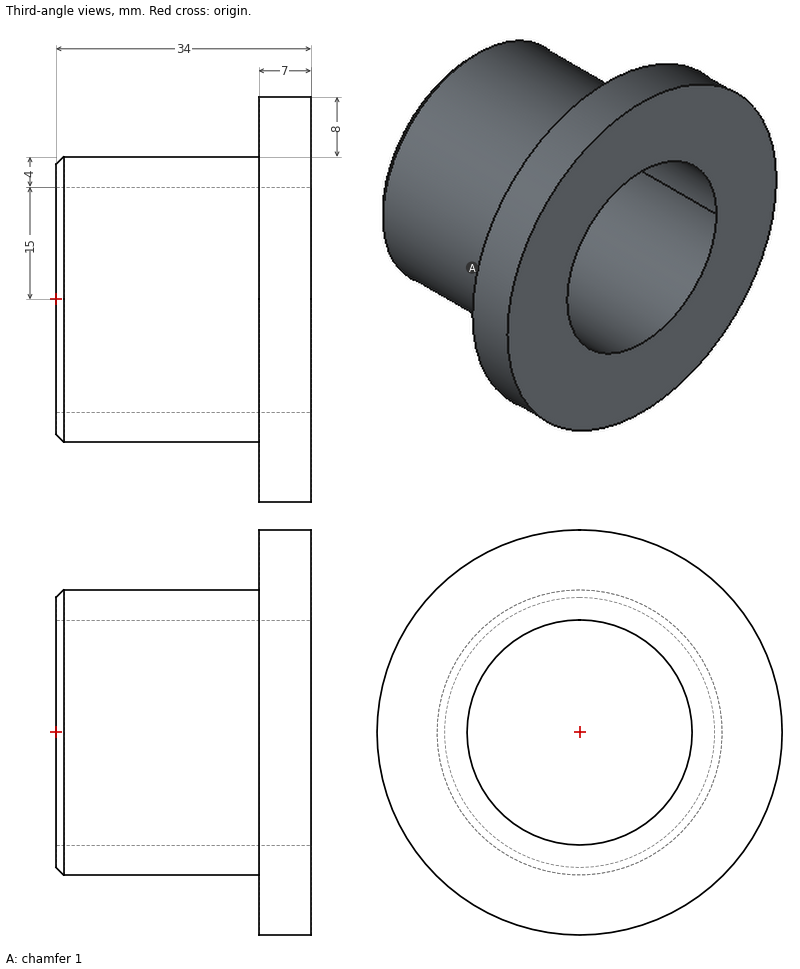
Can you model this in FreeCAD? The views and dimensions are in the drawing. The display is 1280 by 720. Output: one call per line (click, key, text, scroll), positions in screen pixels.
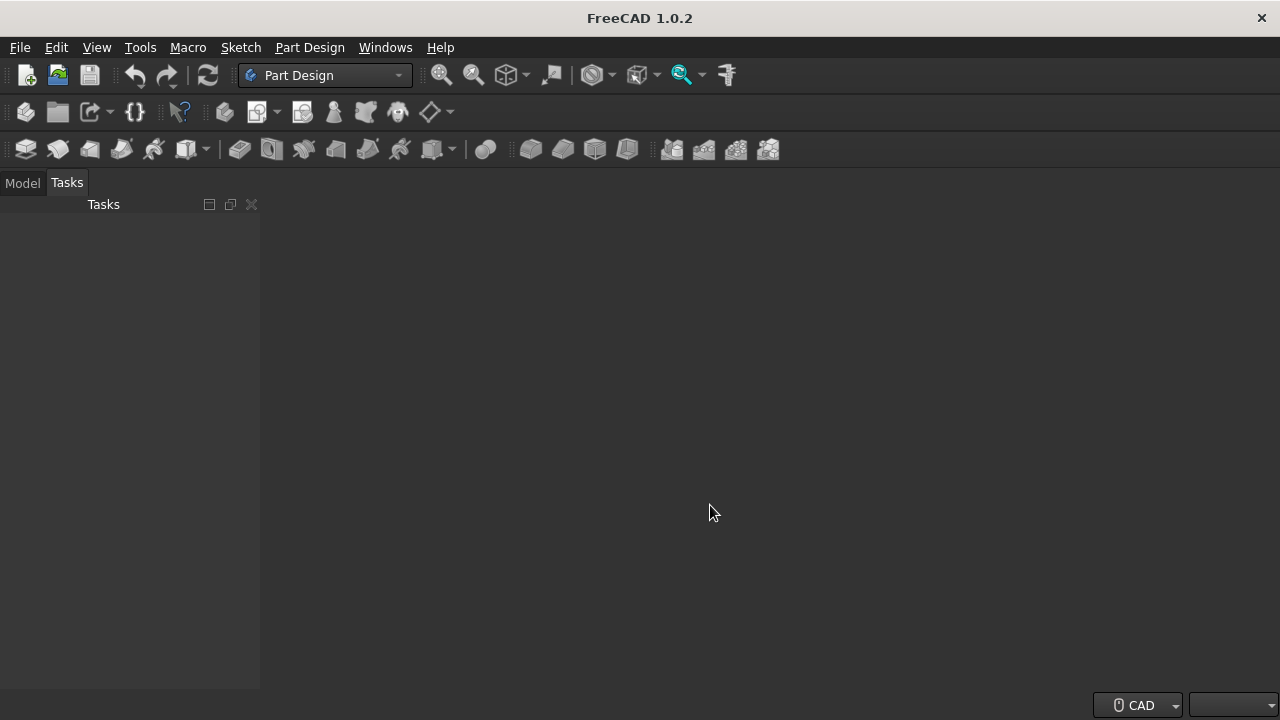
click(26, 76)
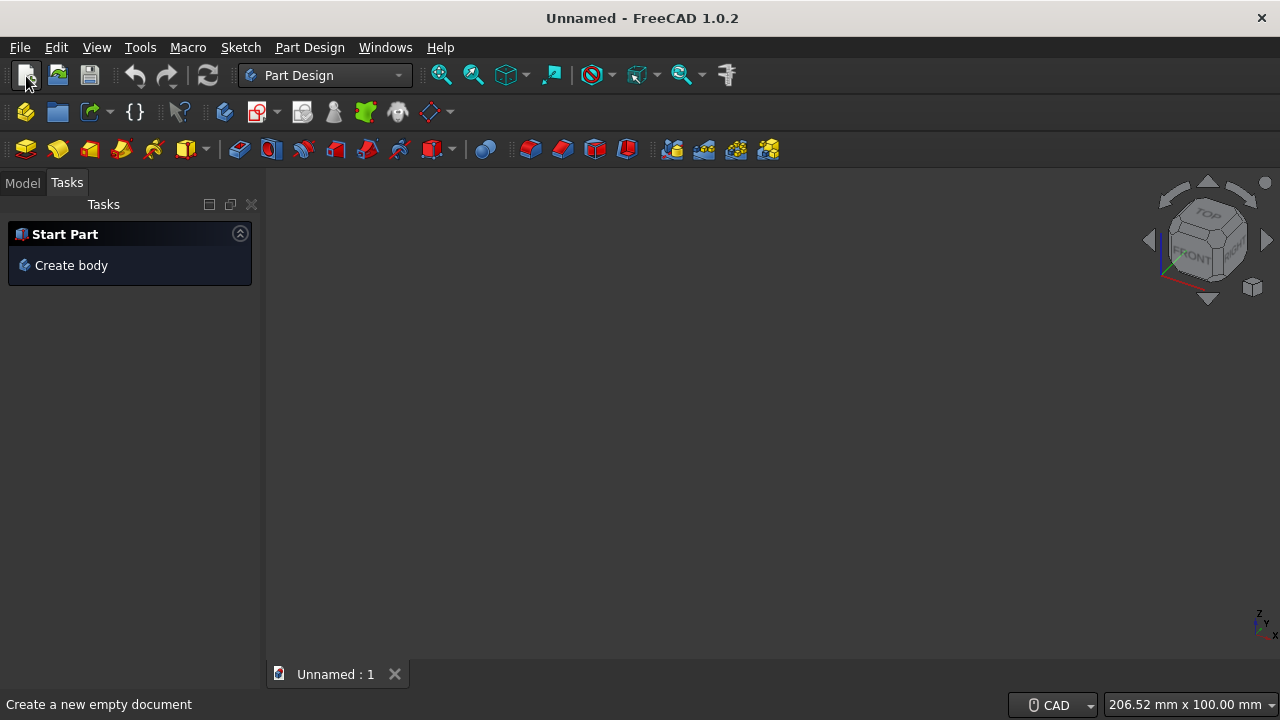
click(258, 112)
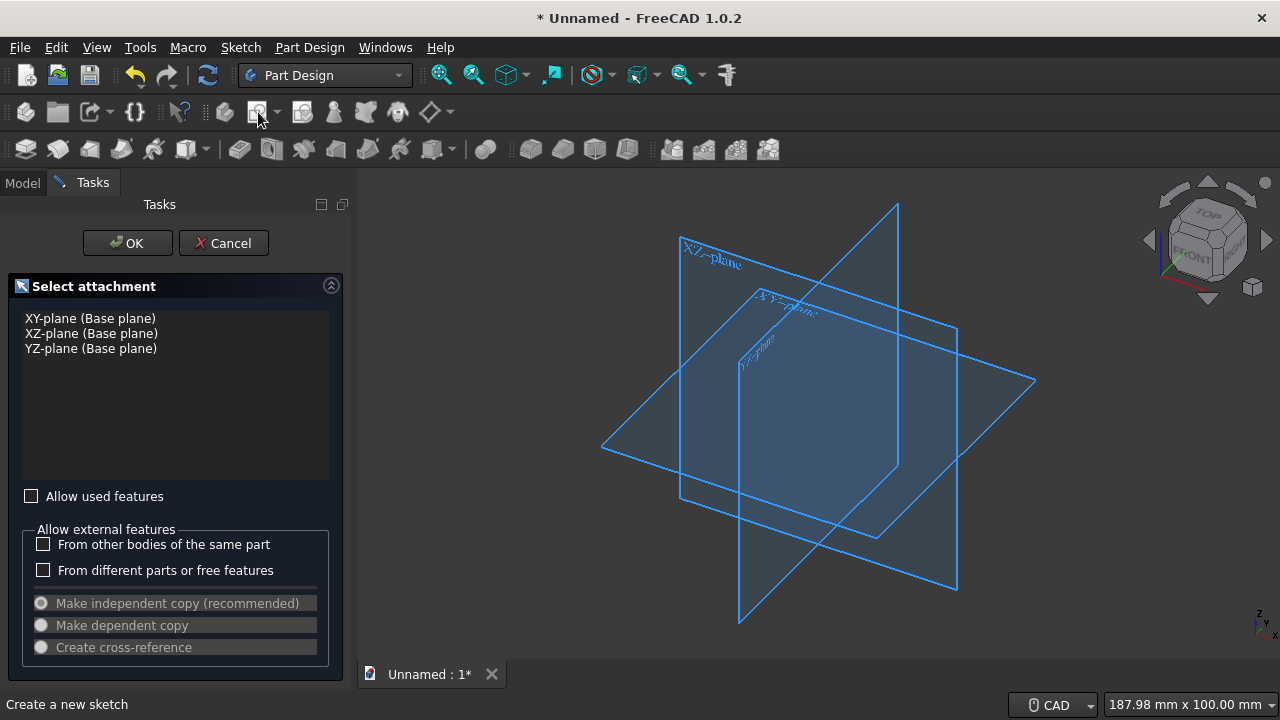
click(82, 318)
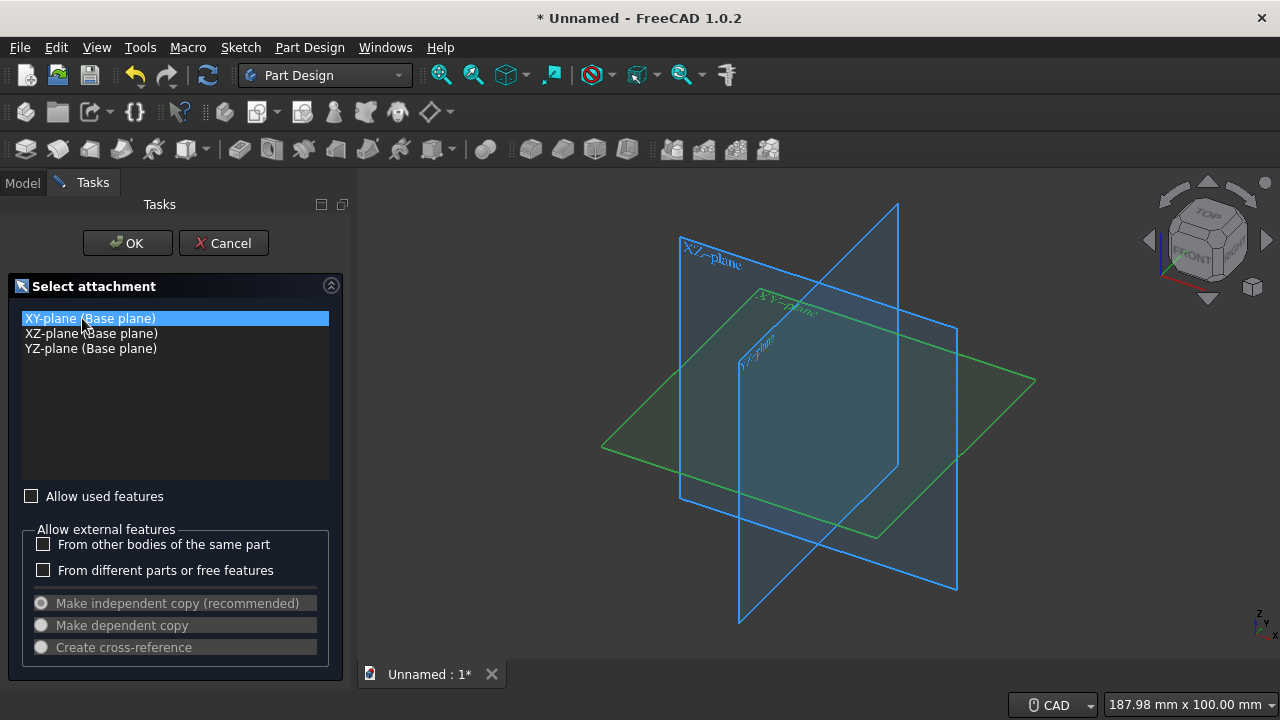
click(128, 243)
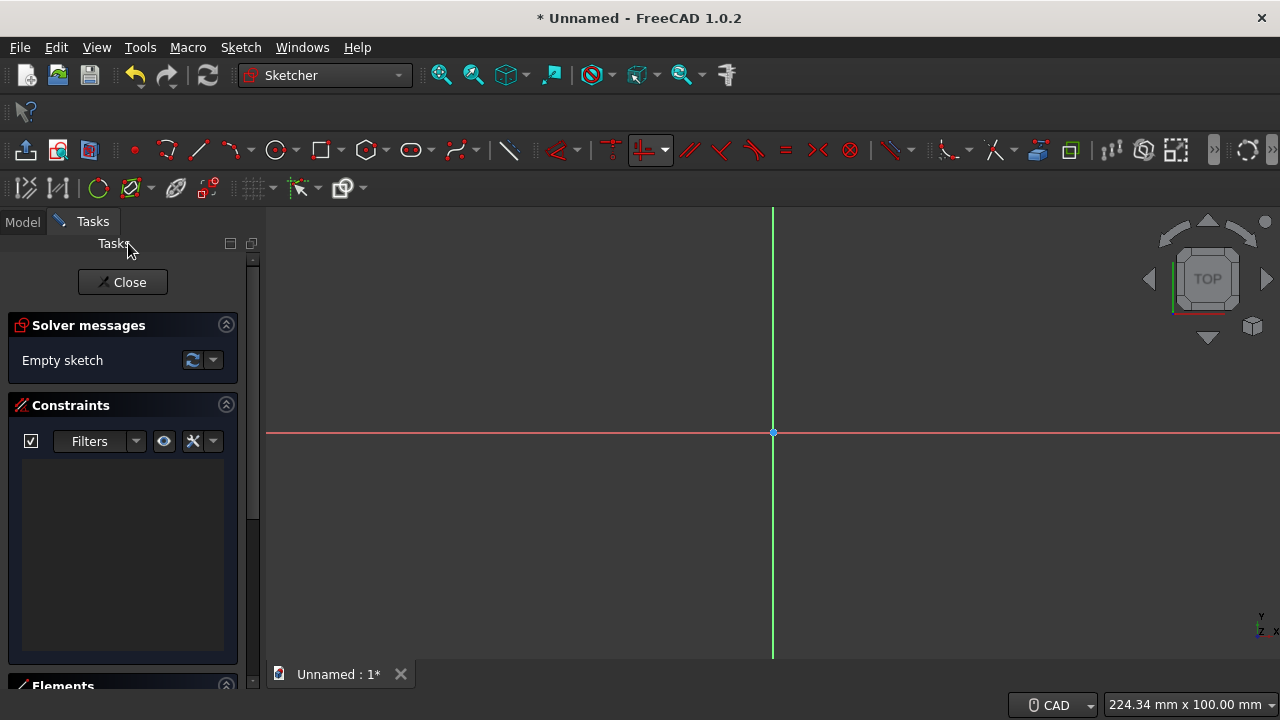
scroll(968, 322, up, 4)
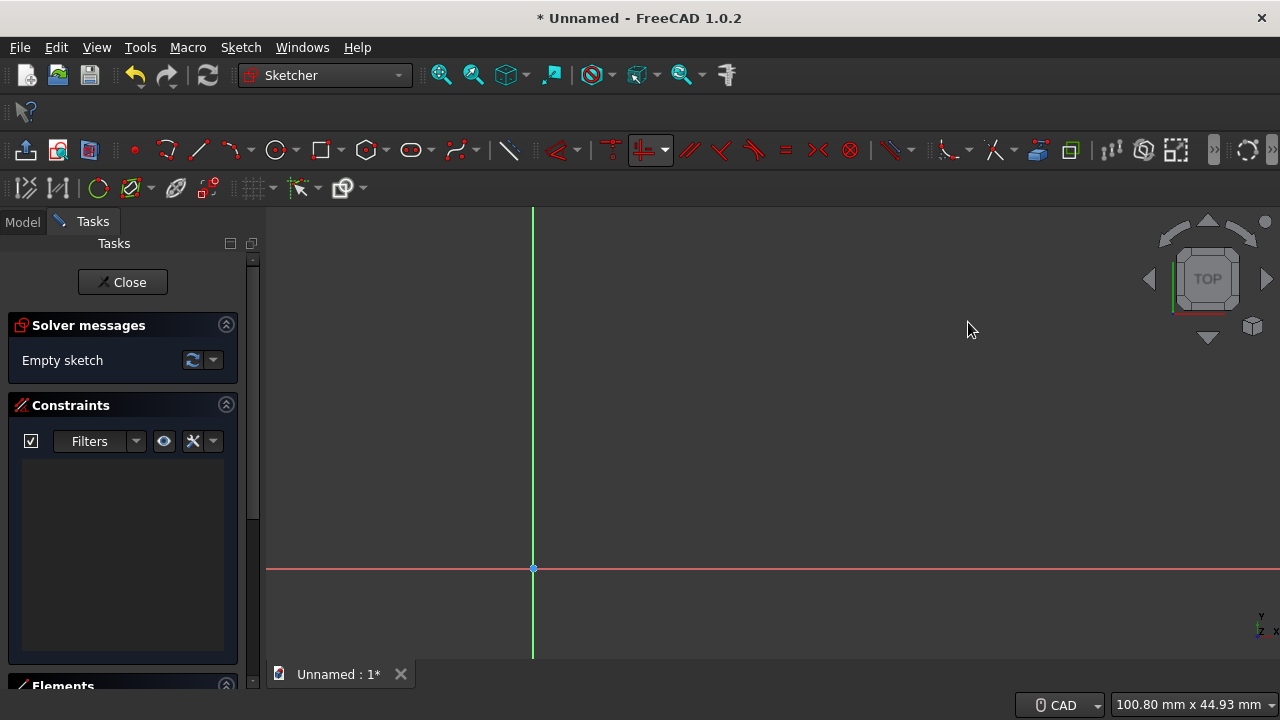
click(168, 150)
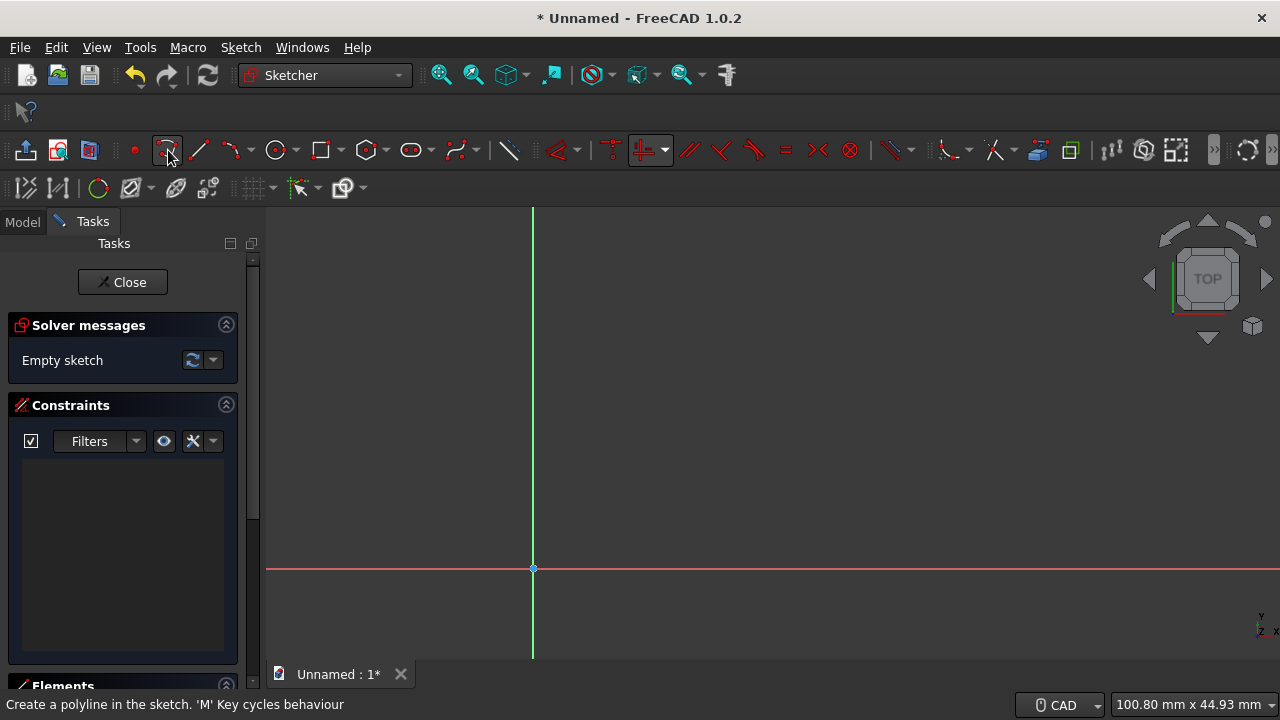
click(533, 418)
click(875, 418)
click(875, 297)
click(805, 297)
click(805, 378)
click(542, 378)
click(533, 419)
key(Escape)
key(Escape)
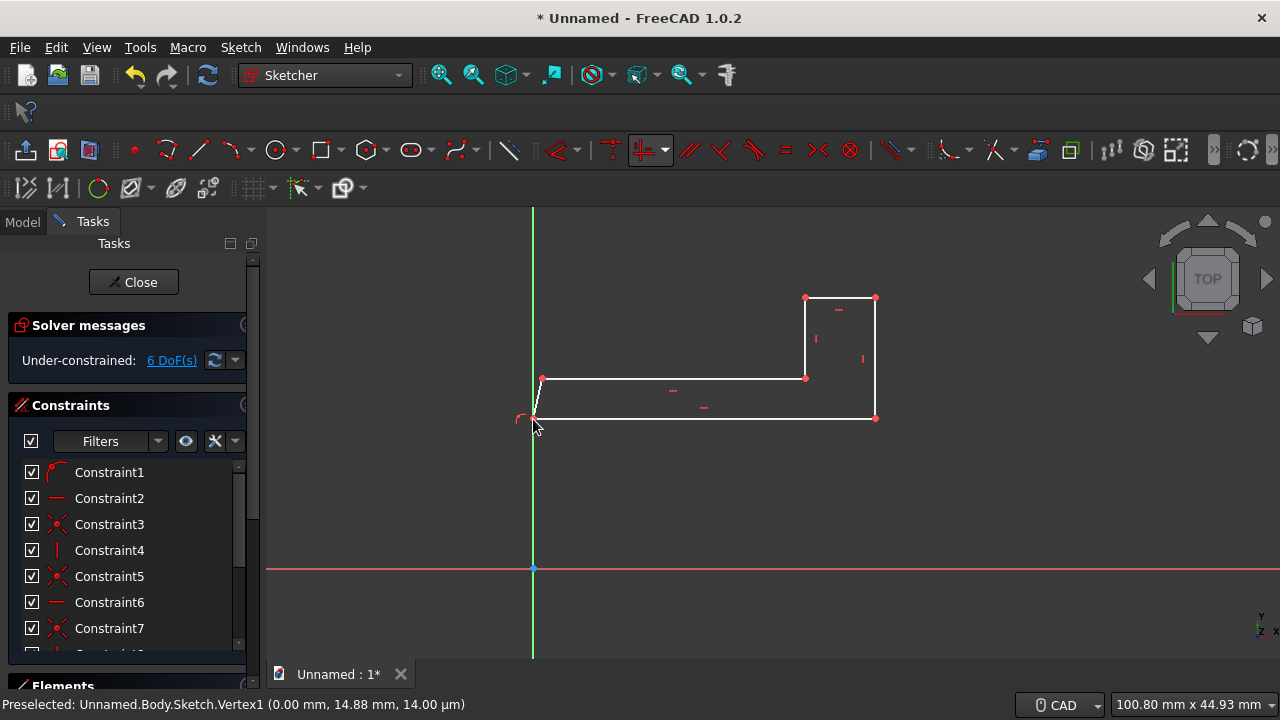
click(536, 407)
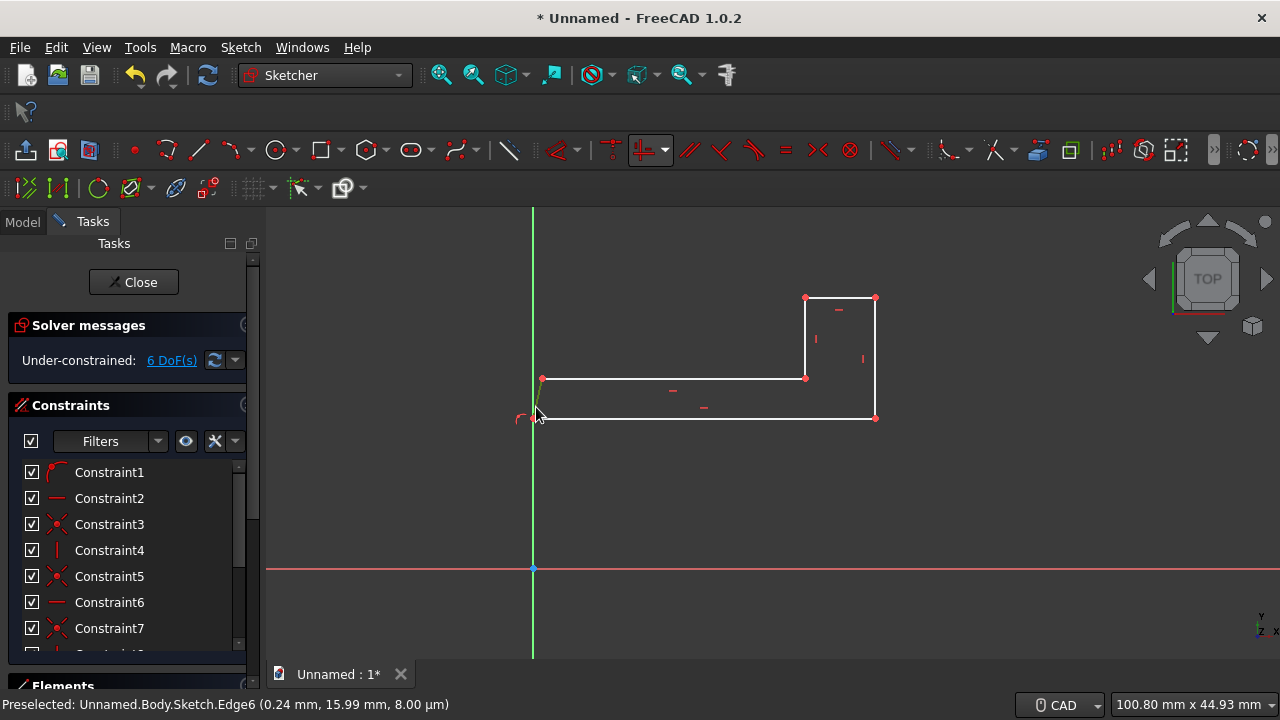
key(v)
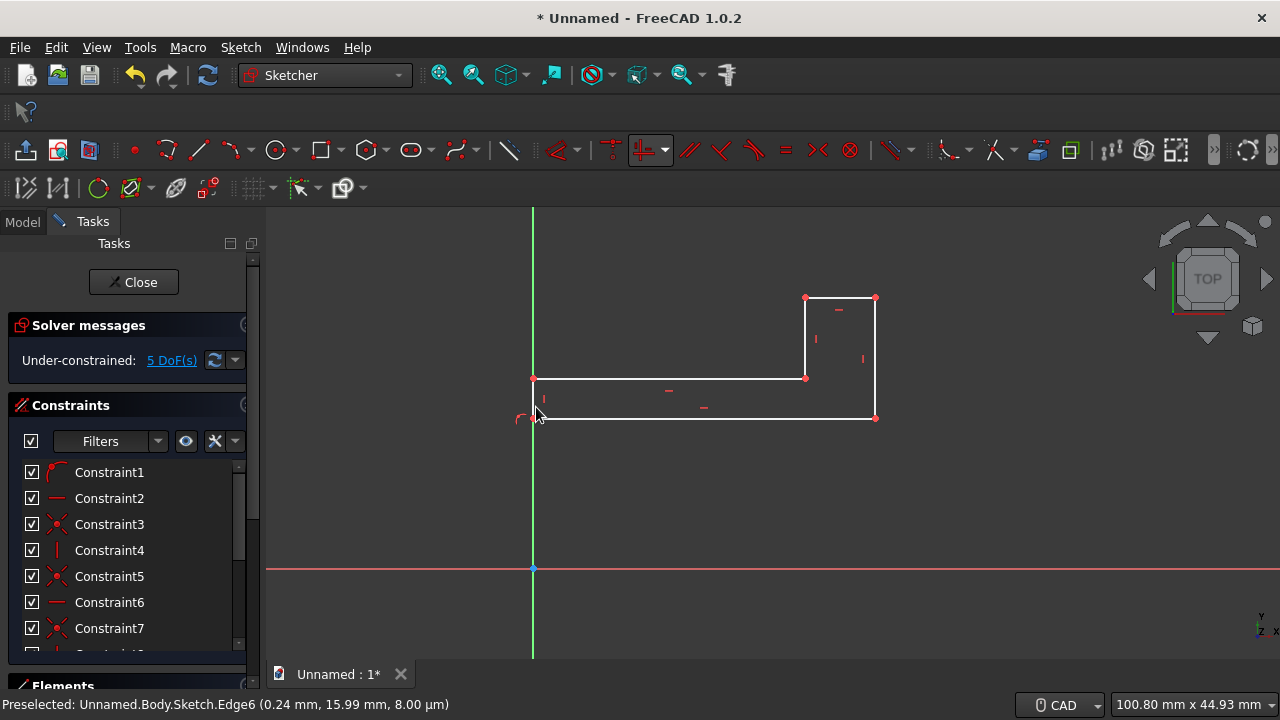
click(854, 298)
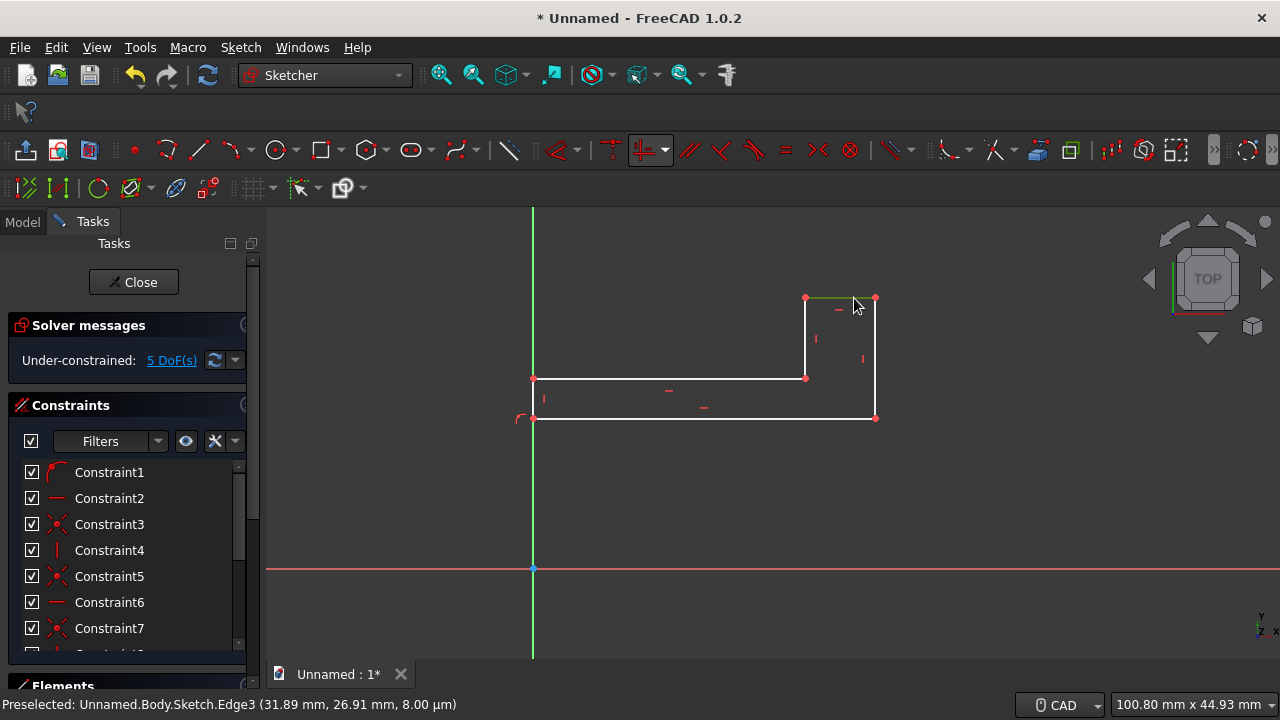
key(l)